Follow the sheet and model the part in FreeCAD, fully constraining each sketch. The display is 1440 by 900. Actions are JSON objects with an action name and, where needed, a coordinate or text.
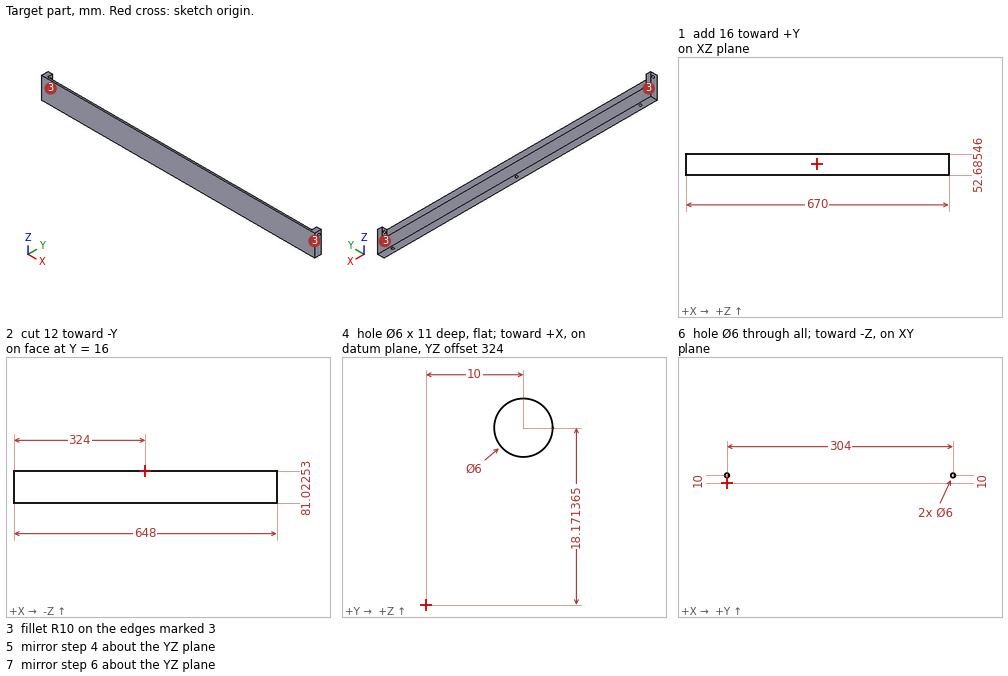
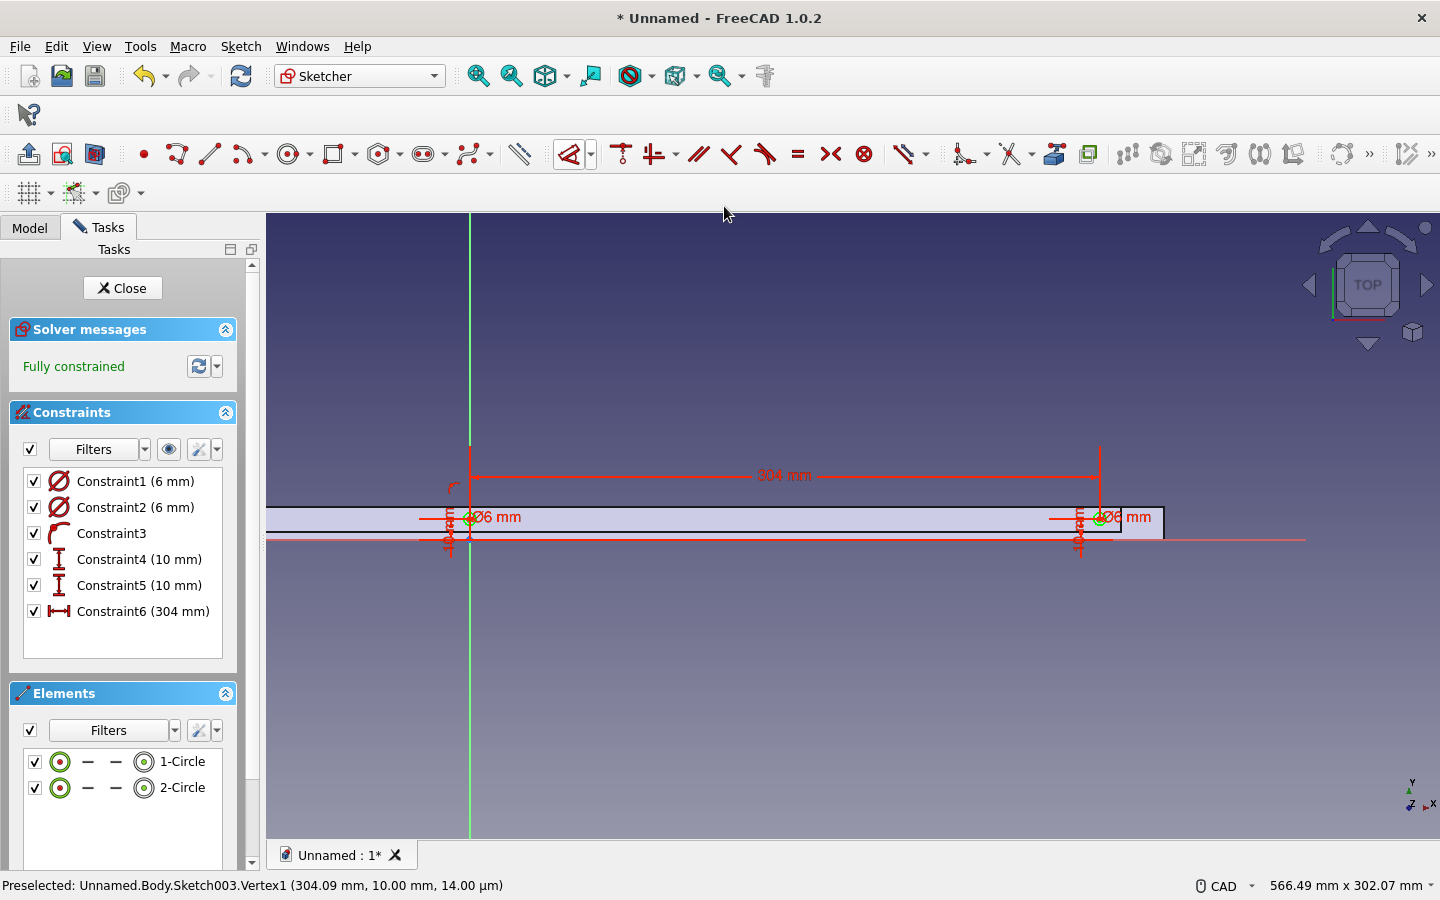
{"action": "left_click", "coordinate": [123, 288]}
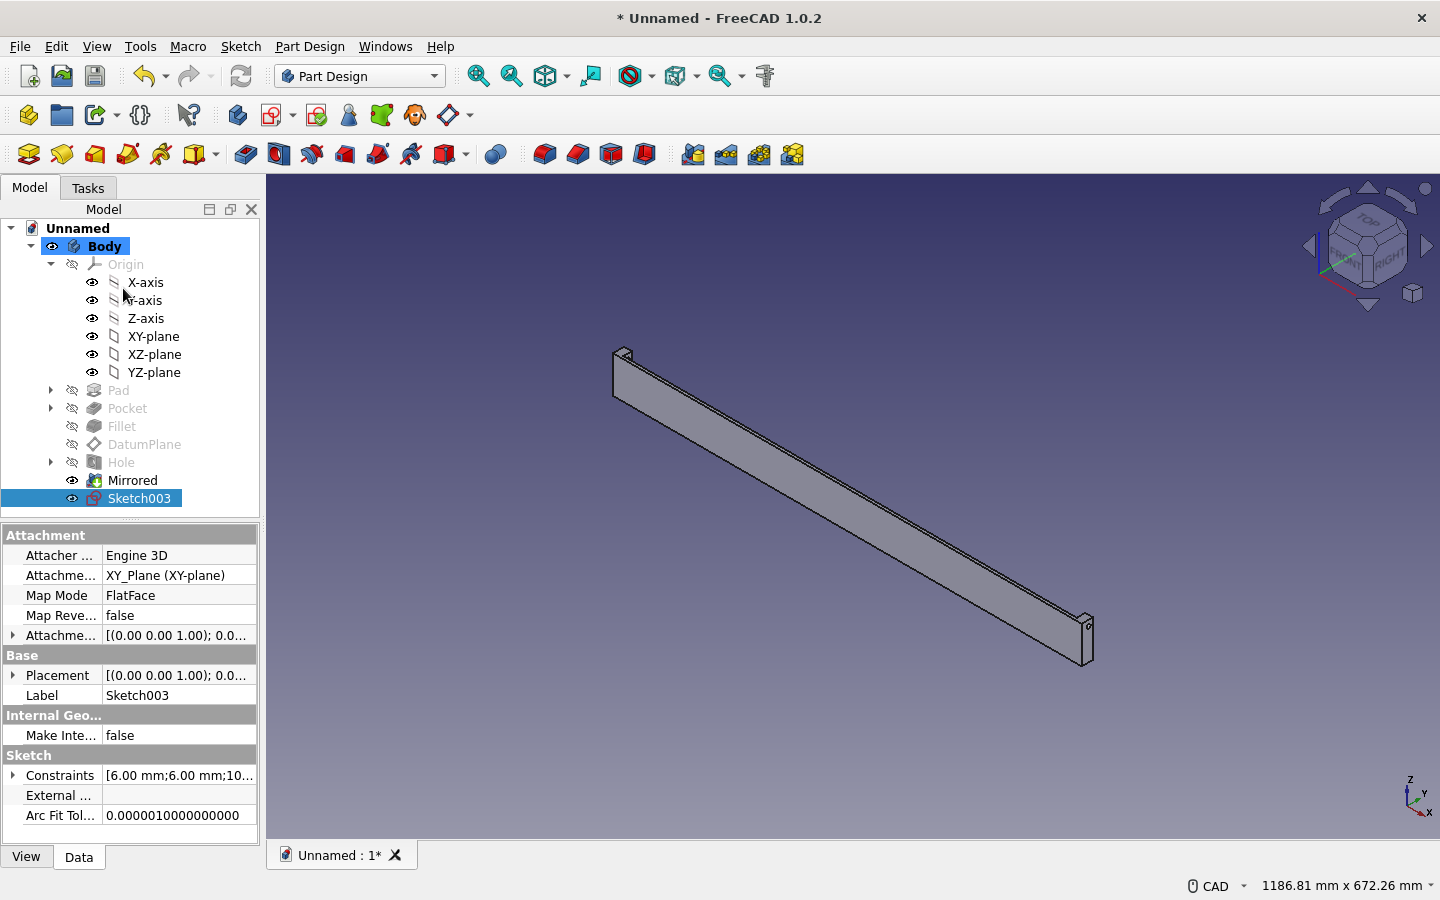
{"action": "left_click", "coordinate": [279, 154]}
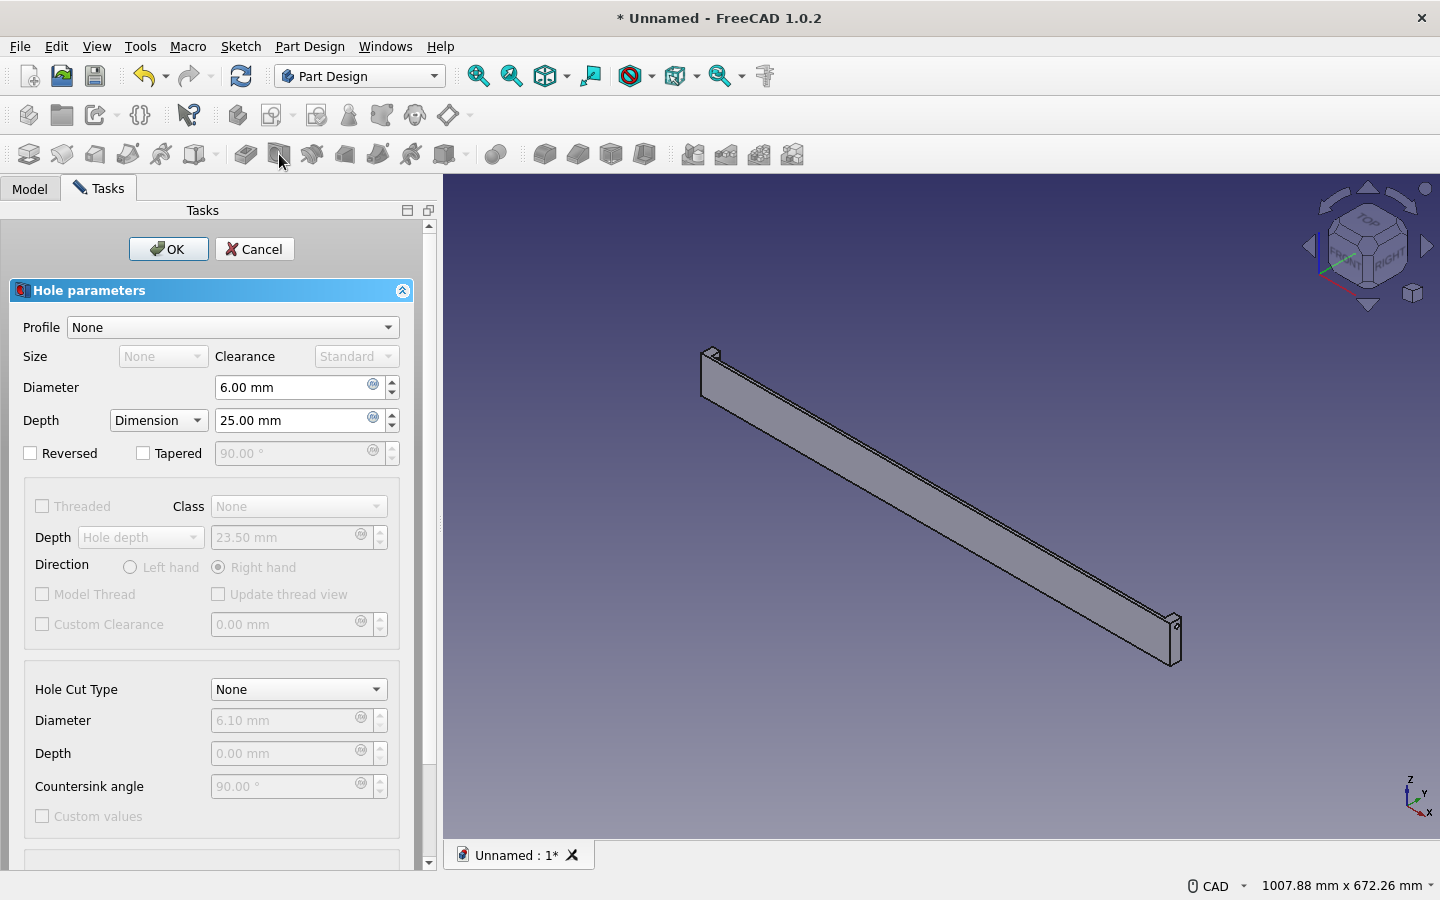
{"action": "triple_click", "coordinate": [300, 388]}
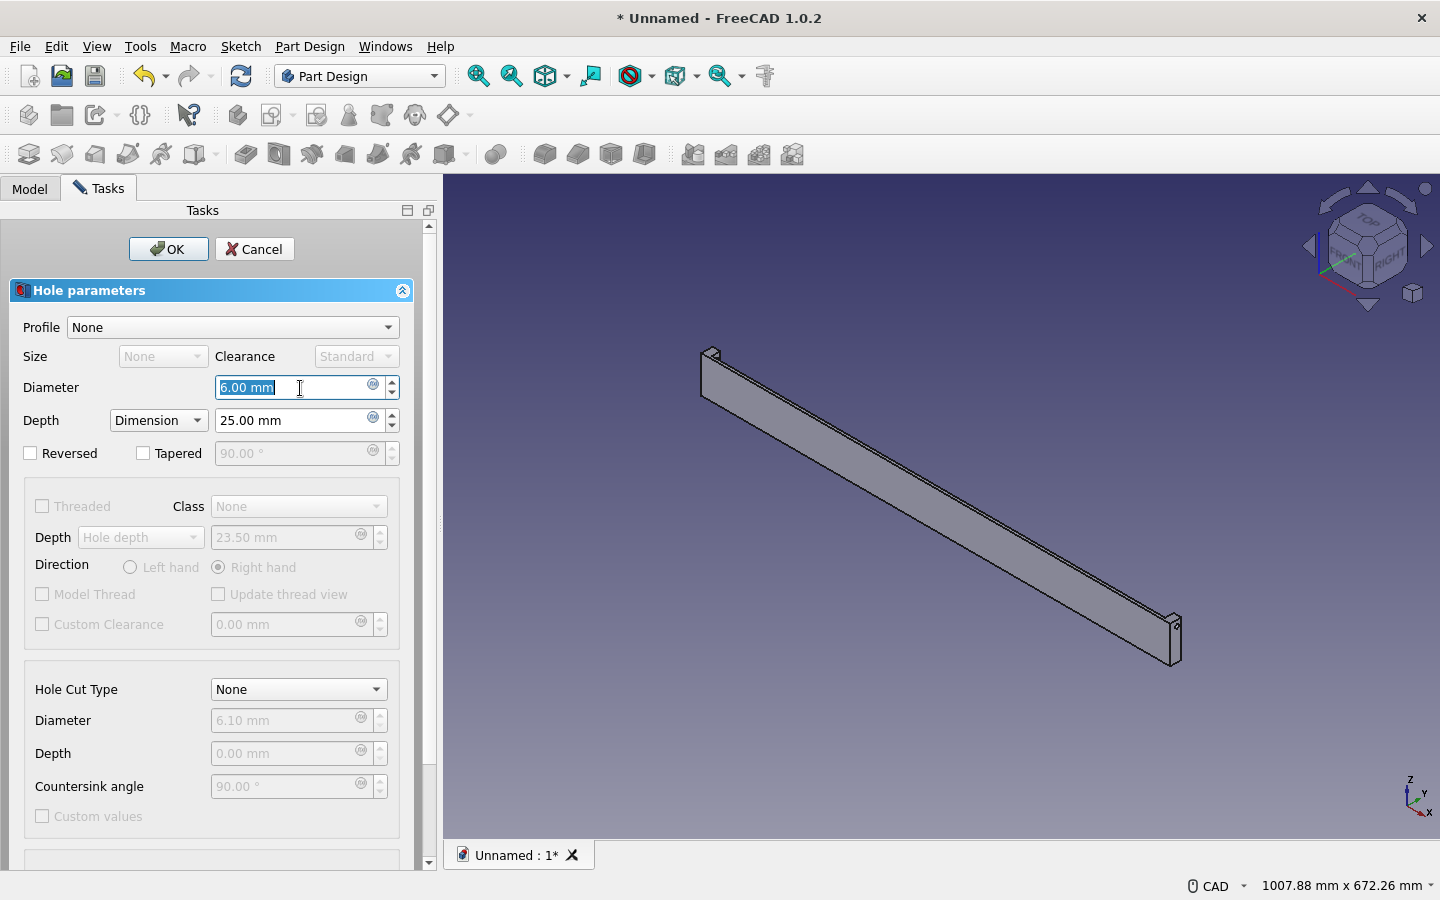
{"action": "type", "text": "6"}
{"action": "key", "text": "Tab"}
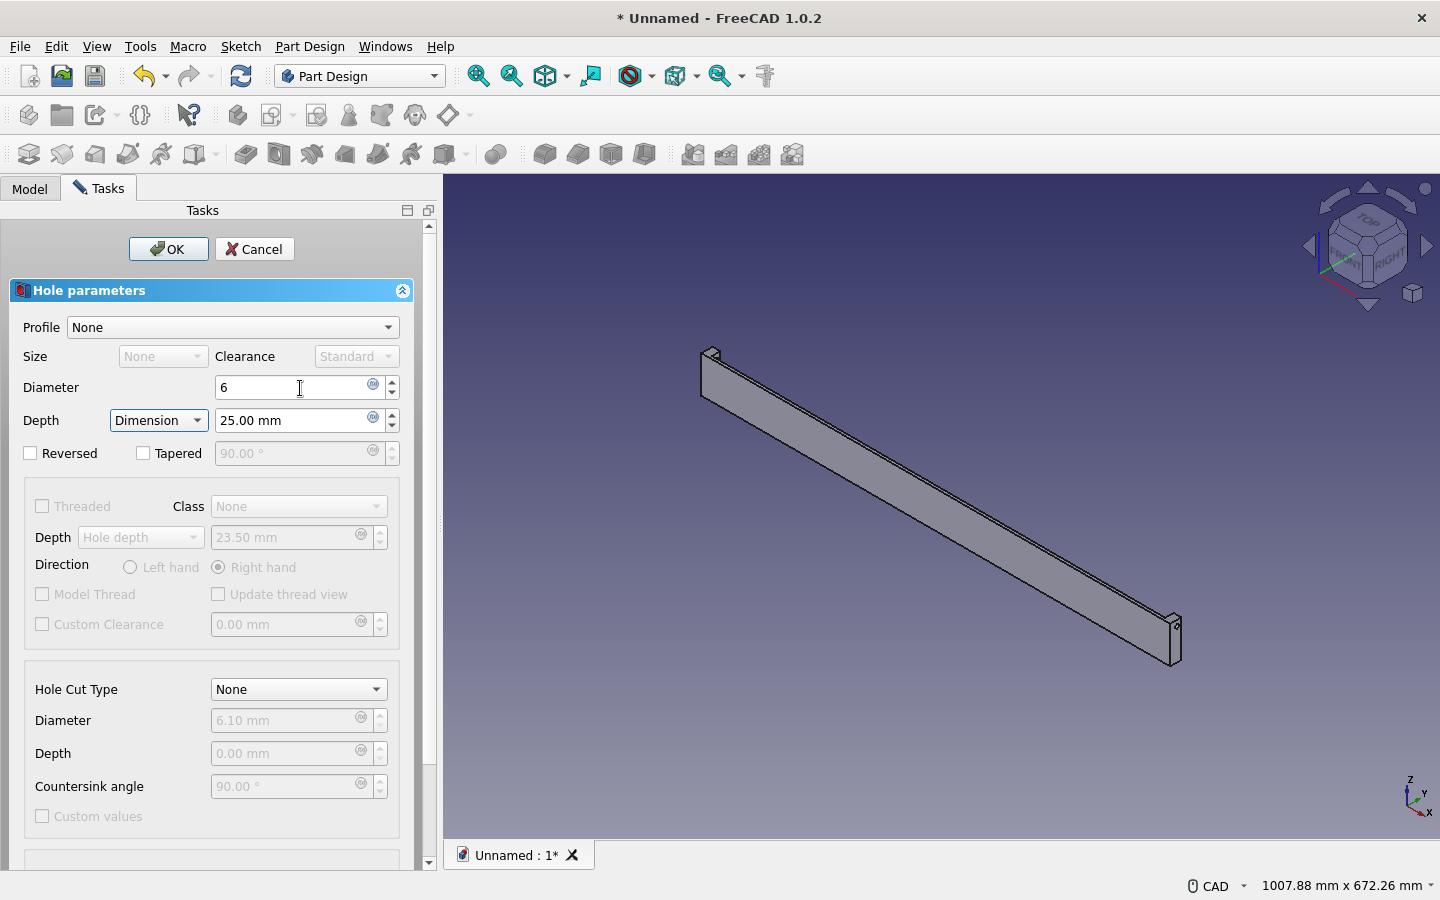
{"action": "left_click", "coordinate": [160, 420]}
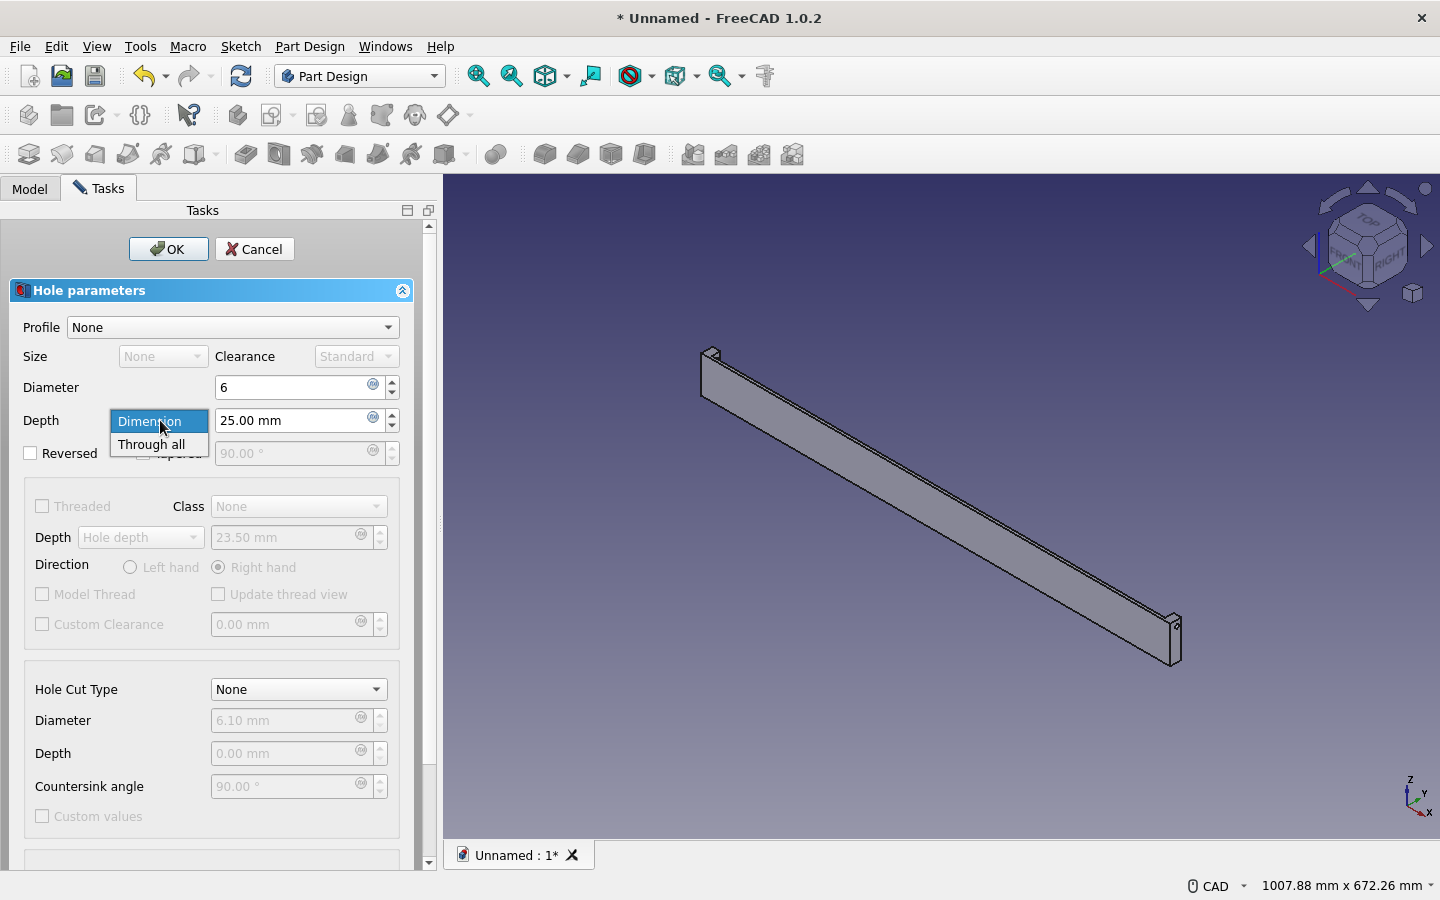
{"action": "left_click", "coordinate": [158, 444]}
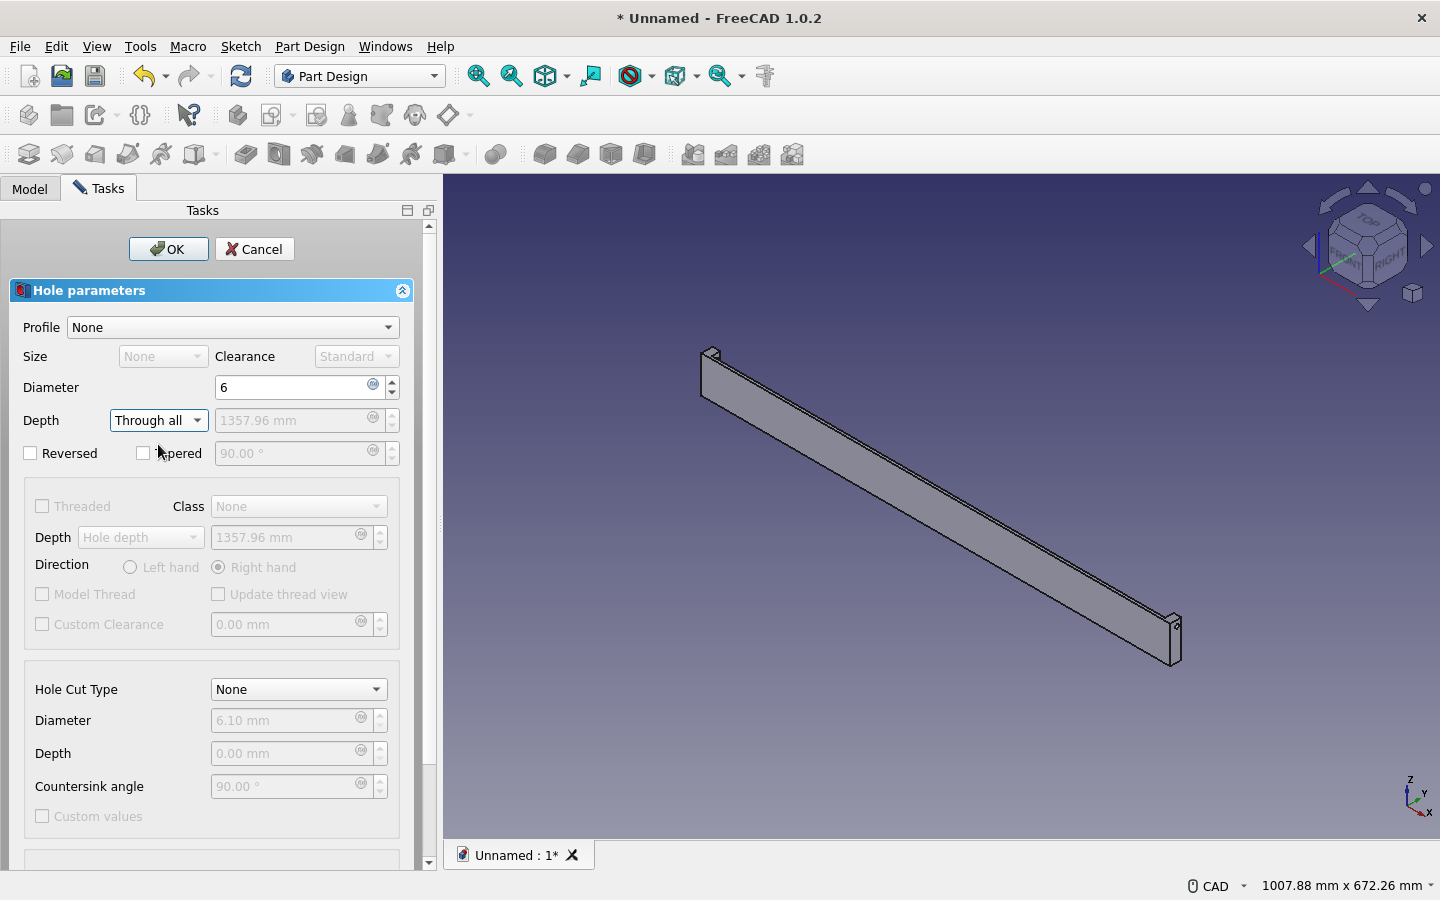
{"action": "left_click", "coordinate": [169, 249]}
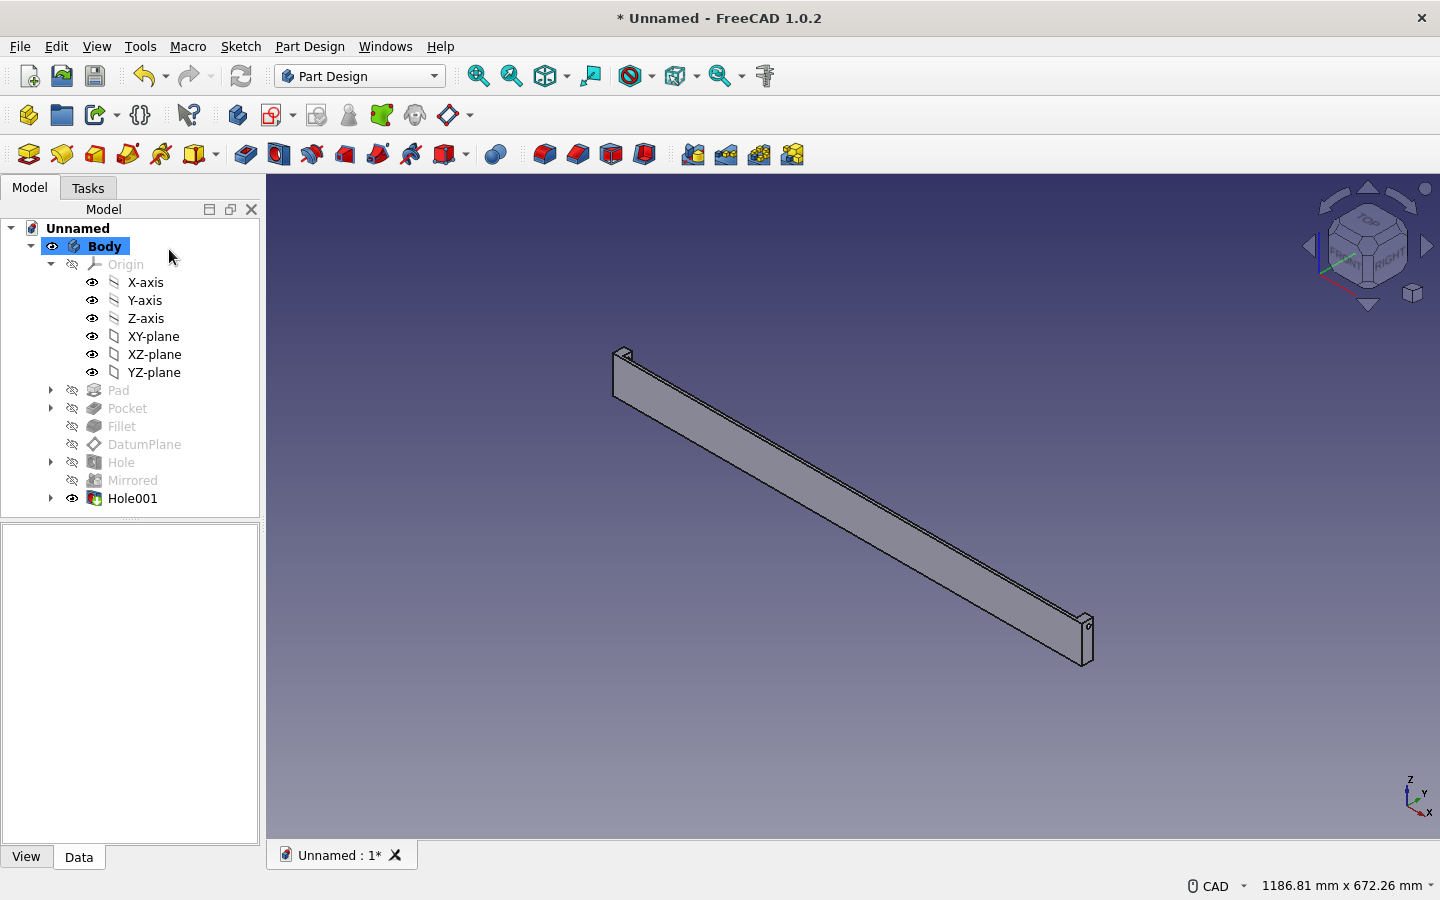
{"action": "left_click", "coordinate": [117, 498]}